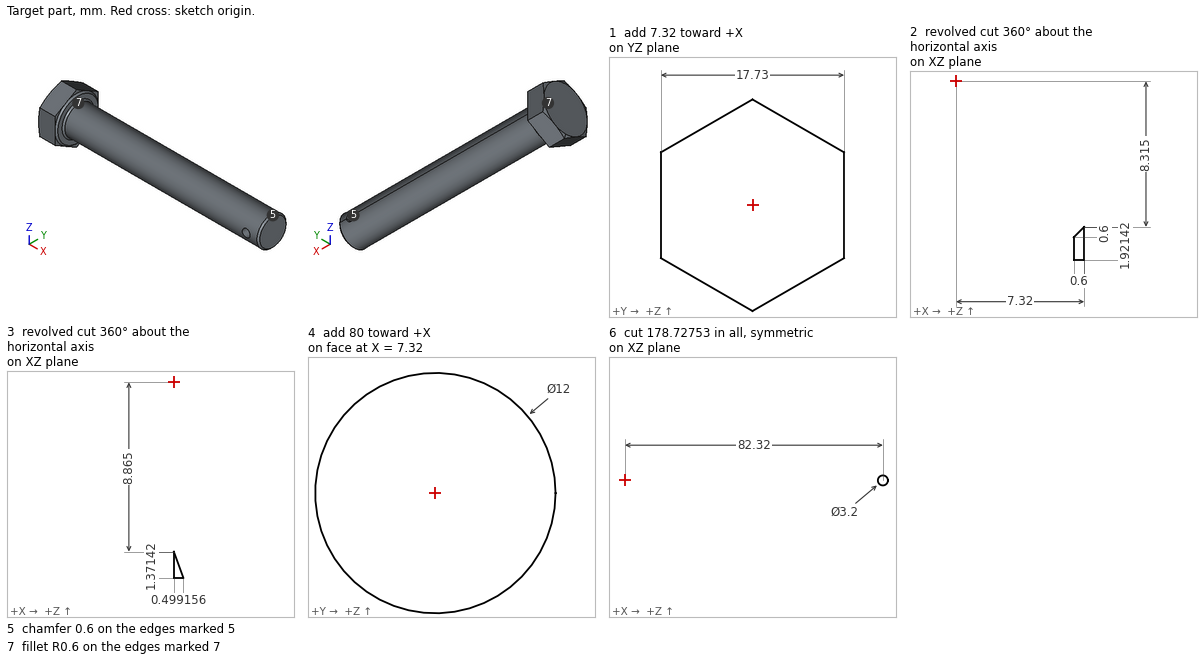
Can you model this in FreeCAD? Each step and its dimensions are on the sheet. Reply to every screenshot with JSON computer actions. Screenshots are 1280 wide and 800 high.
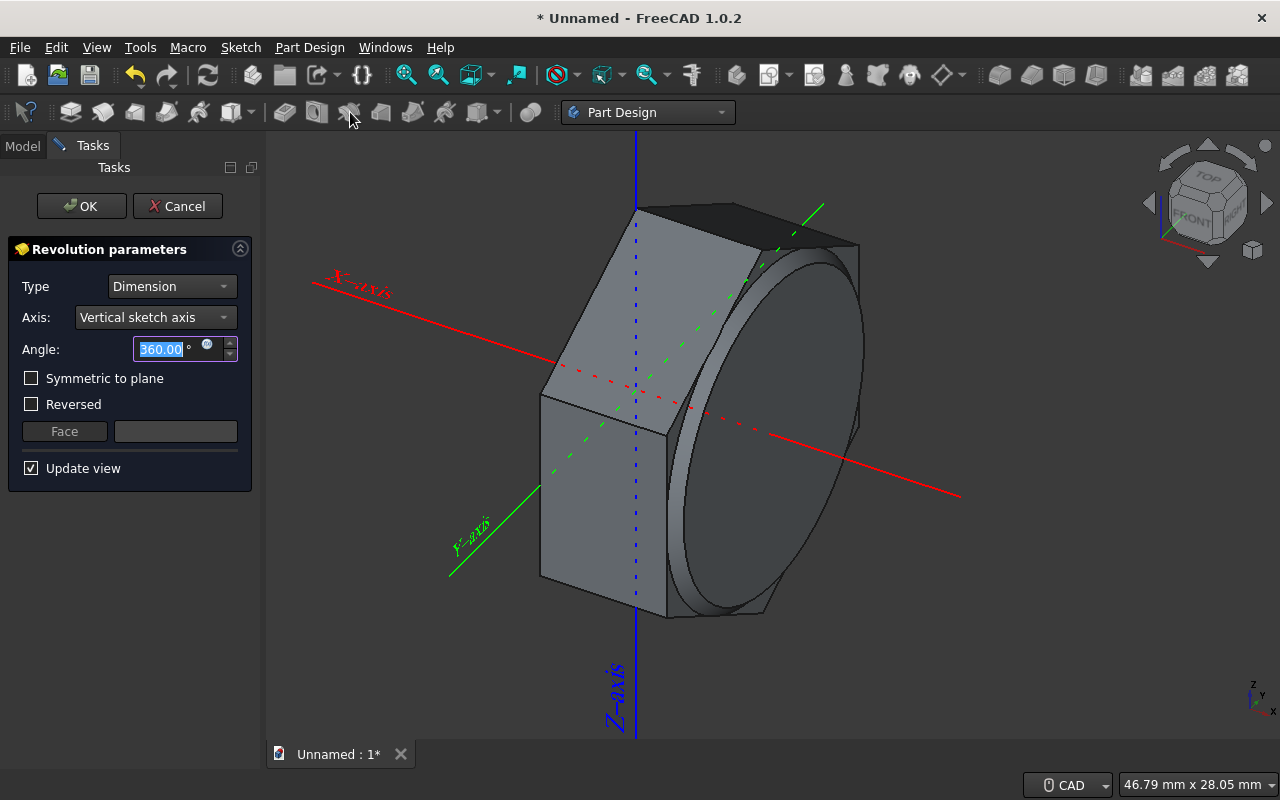
{"action": "left_click", "coordinate": [156, 318]}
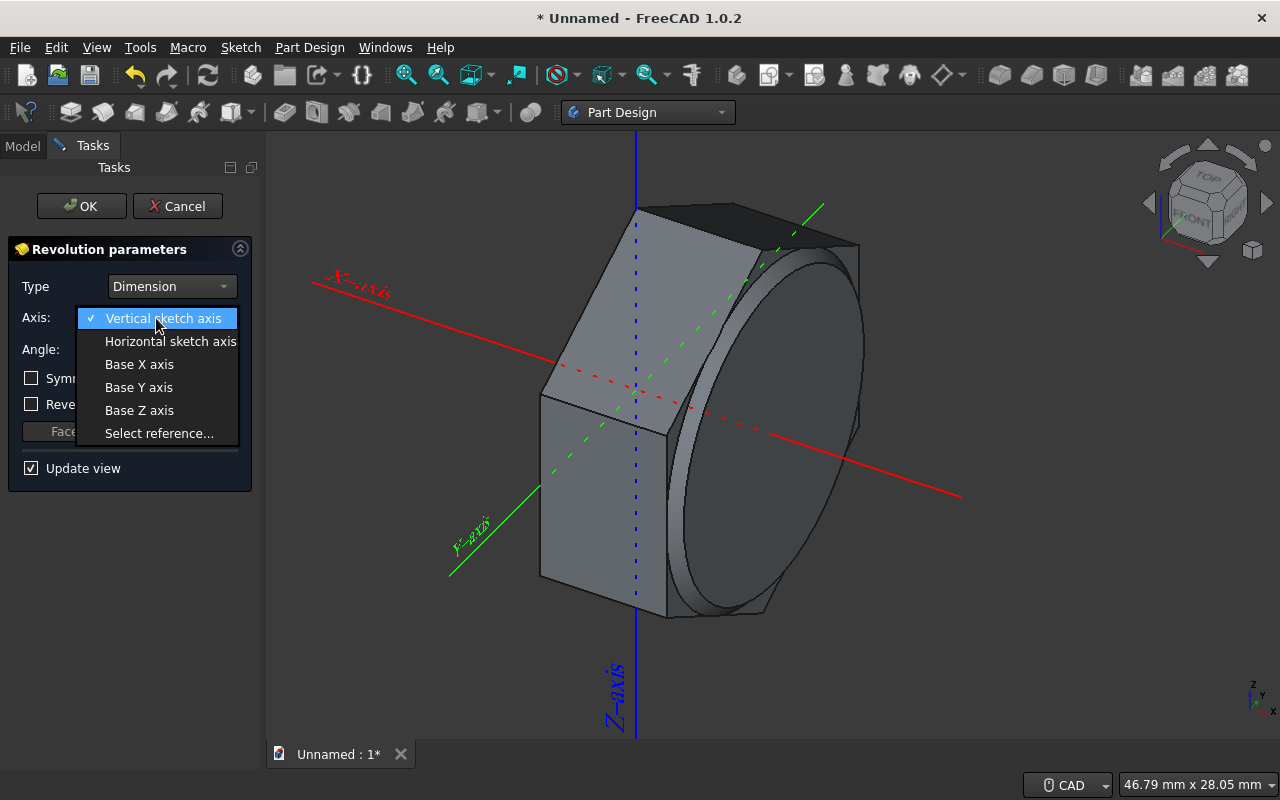
{"action": "left_click", "coordinate": [156, 342]}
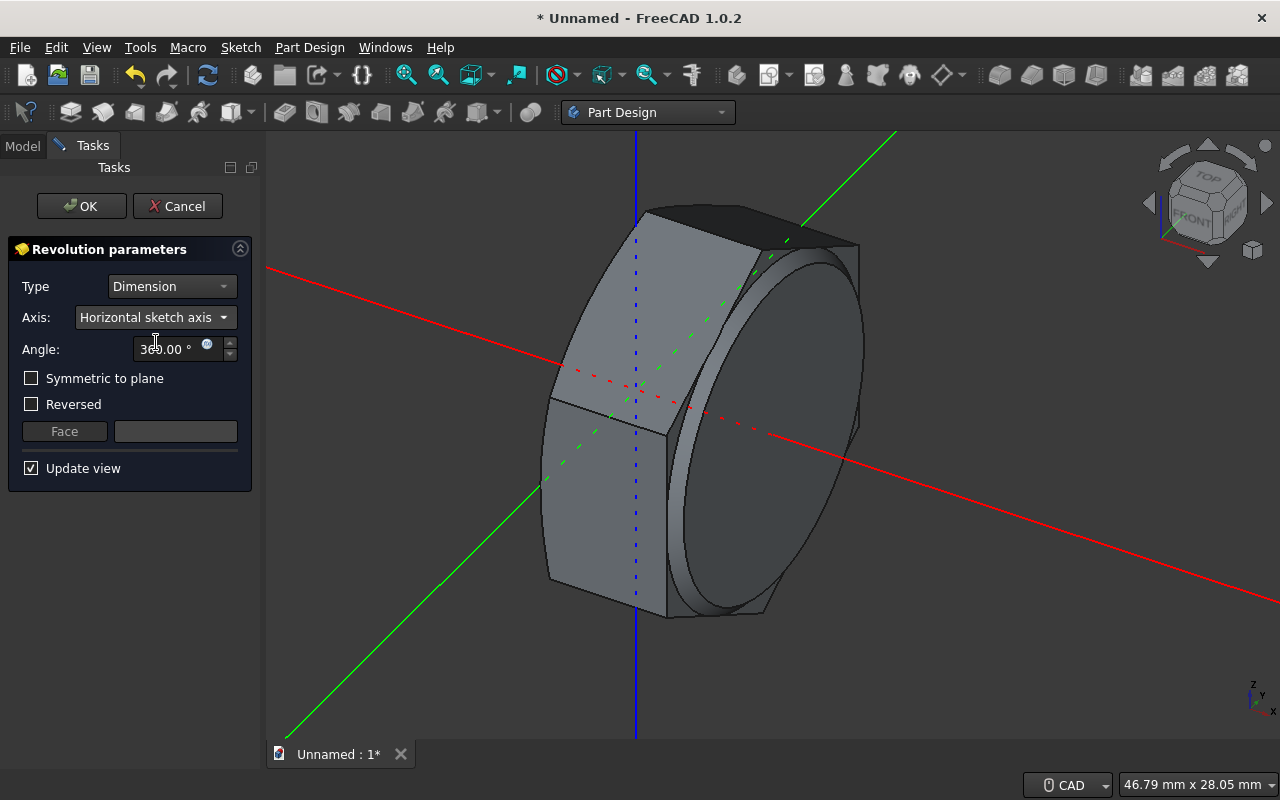
{"action": "left_click", "coordinate": [82, 206]}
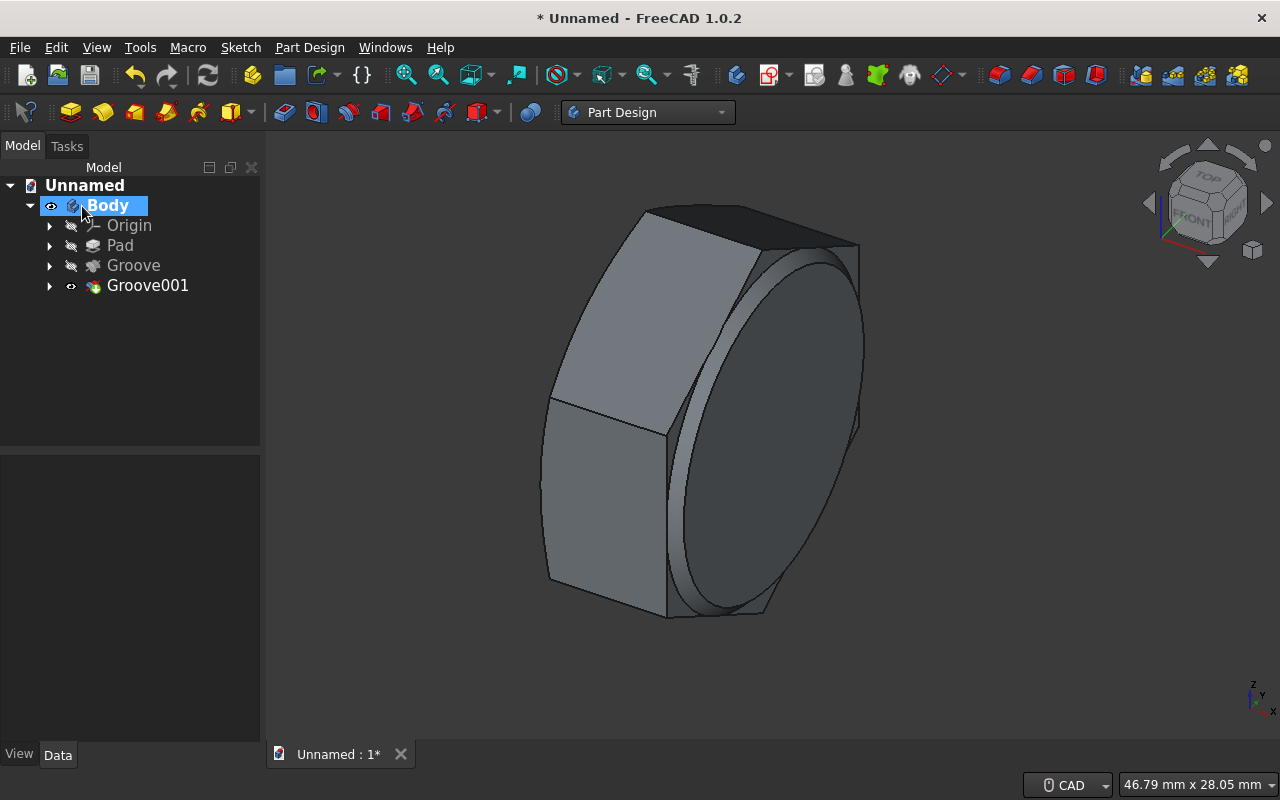
{"action": "left_click", "coordinate": [408, 76]}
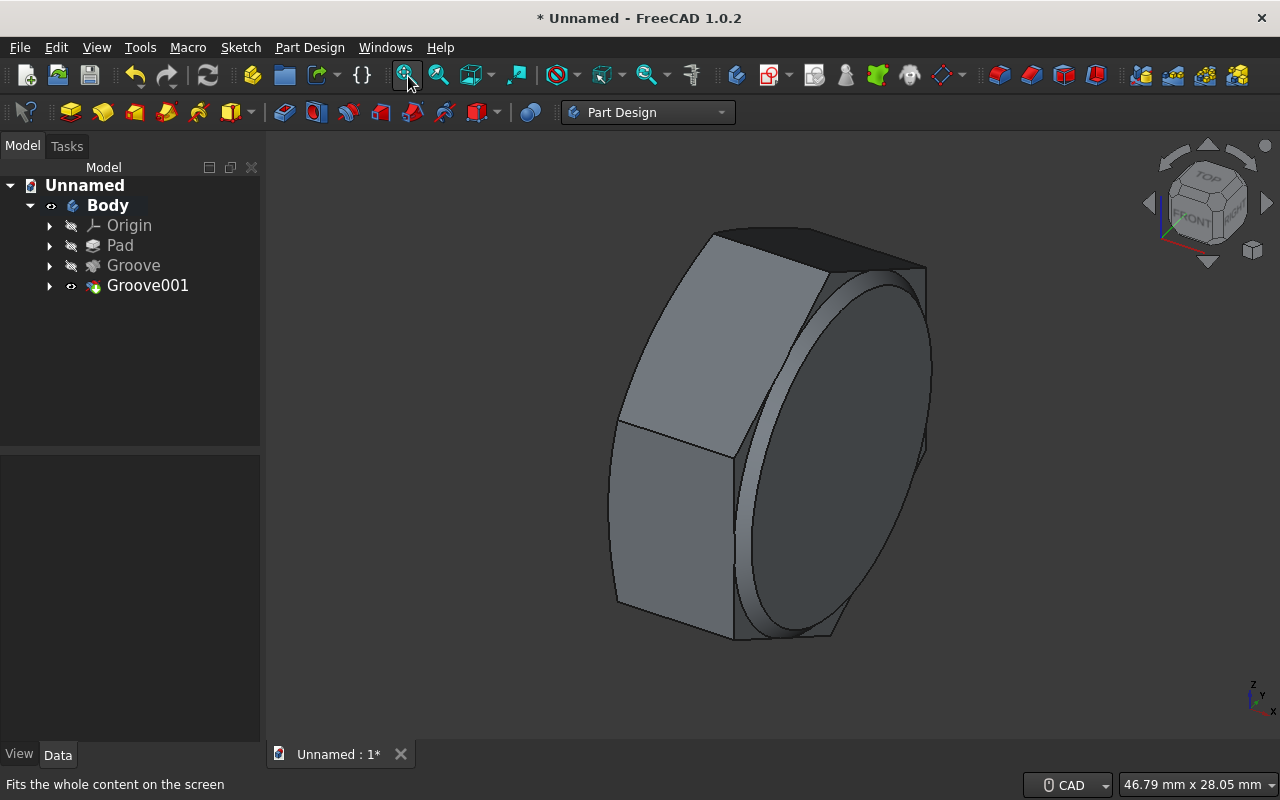
{"action": "left_click", "coordinate": [842, 457]}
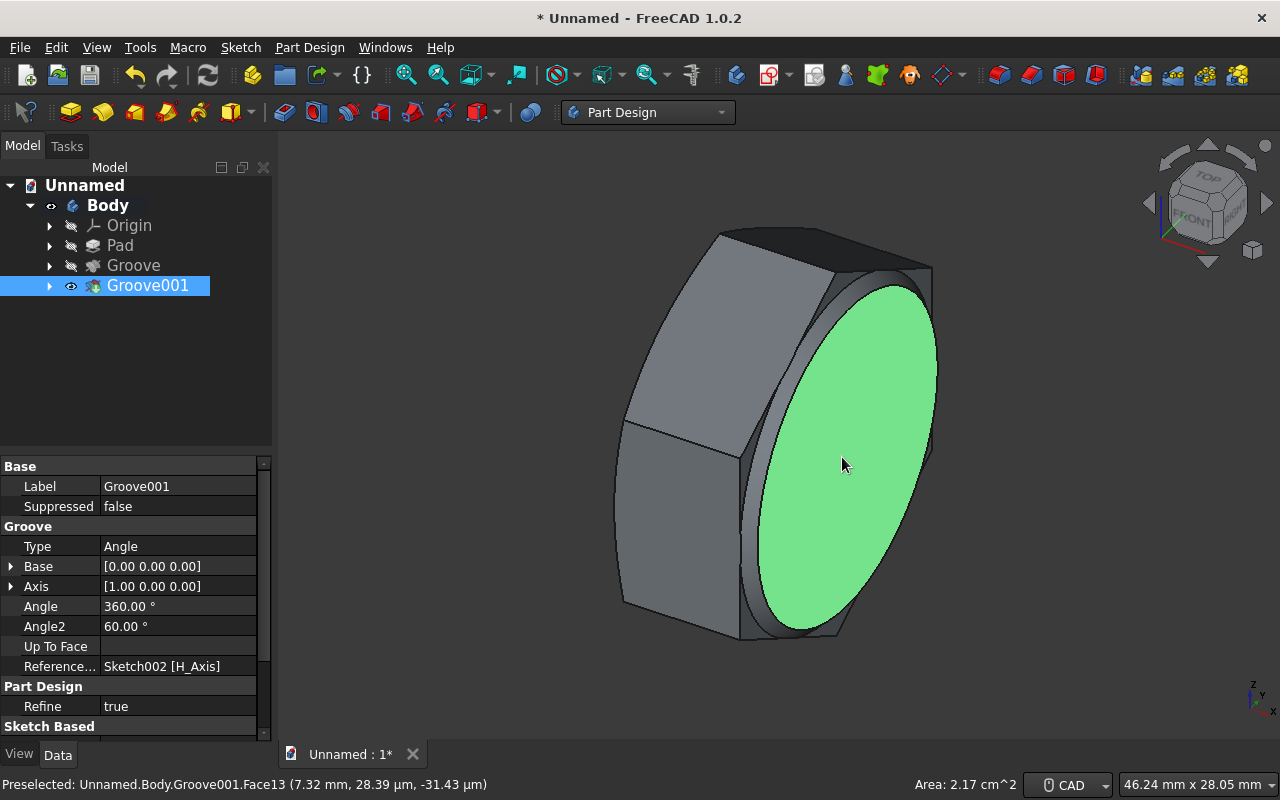
{"action": "left_click", "coordinate": [770, 76]}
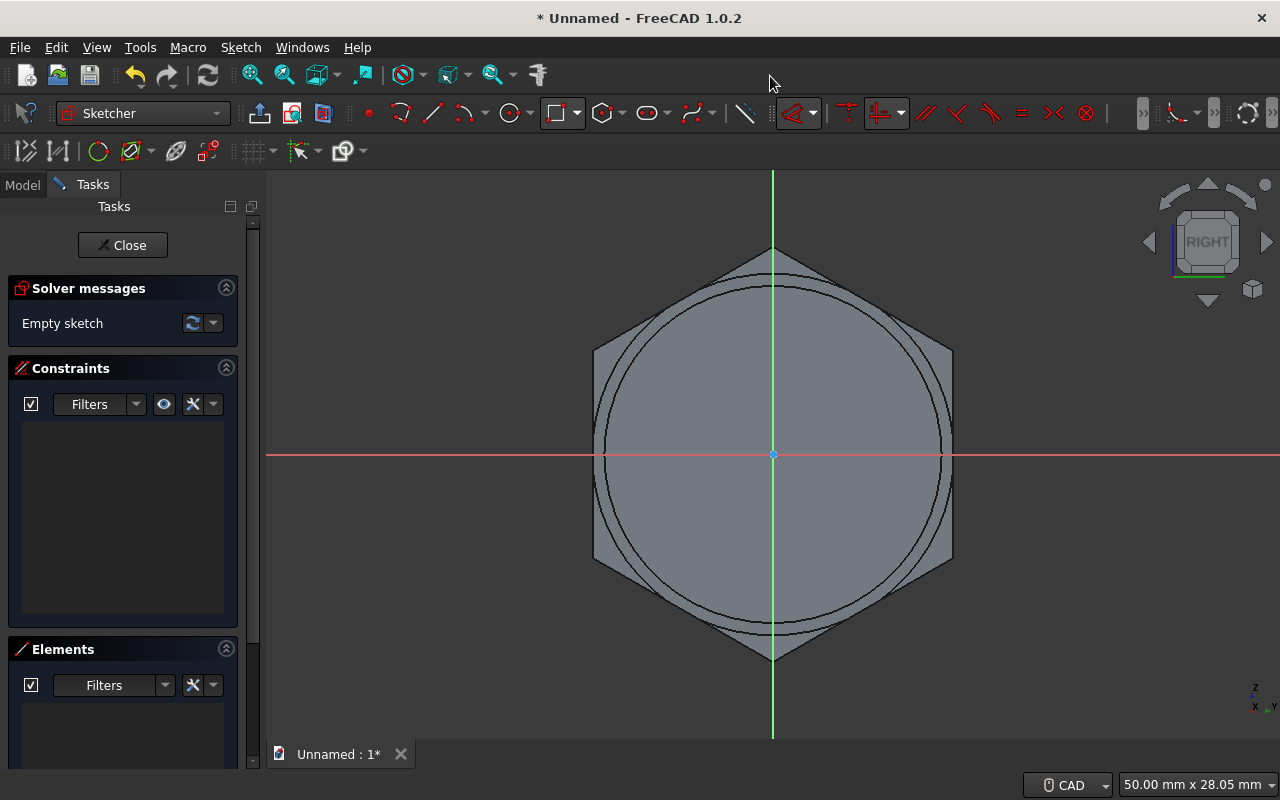
{"action": "scroll", "coordinate": [912, 455], "scroll_direction": "up", "scroll_amount": 2}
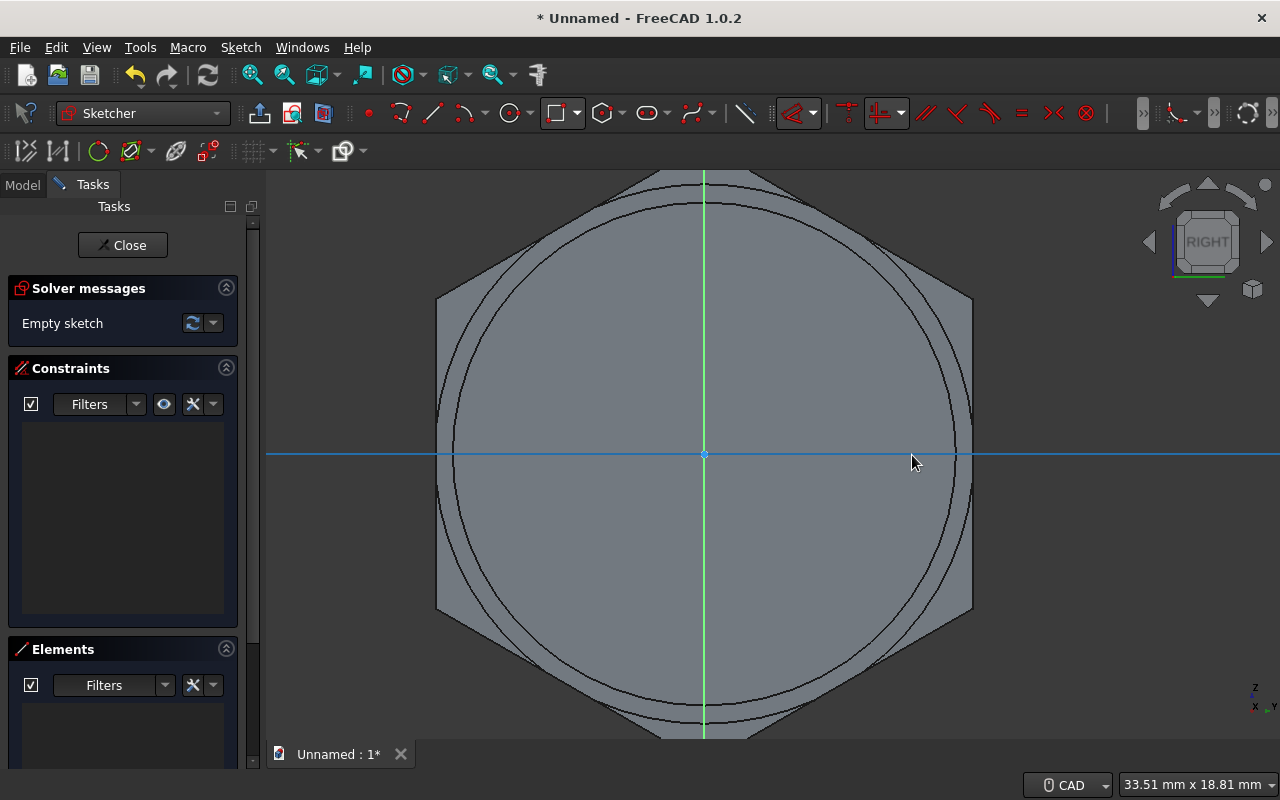
{"action": "left_click", "coordinate": [510, 114]}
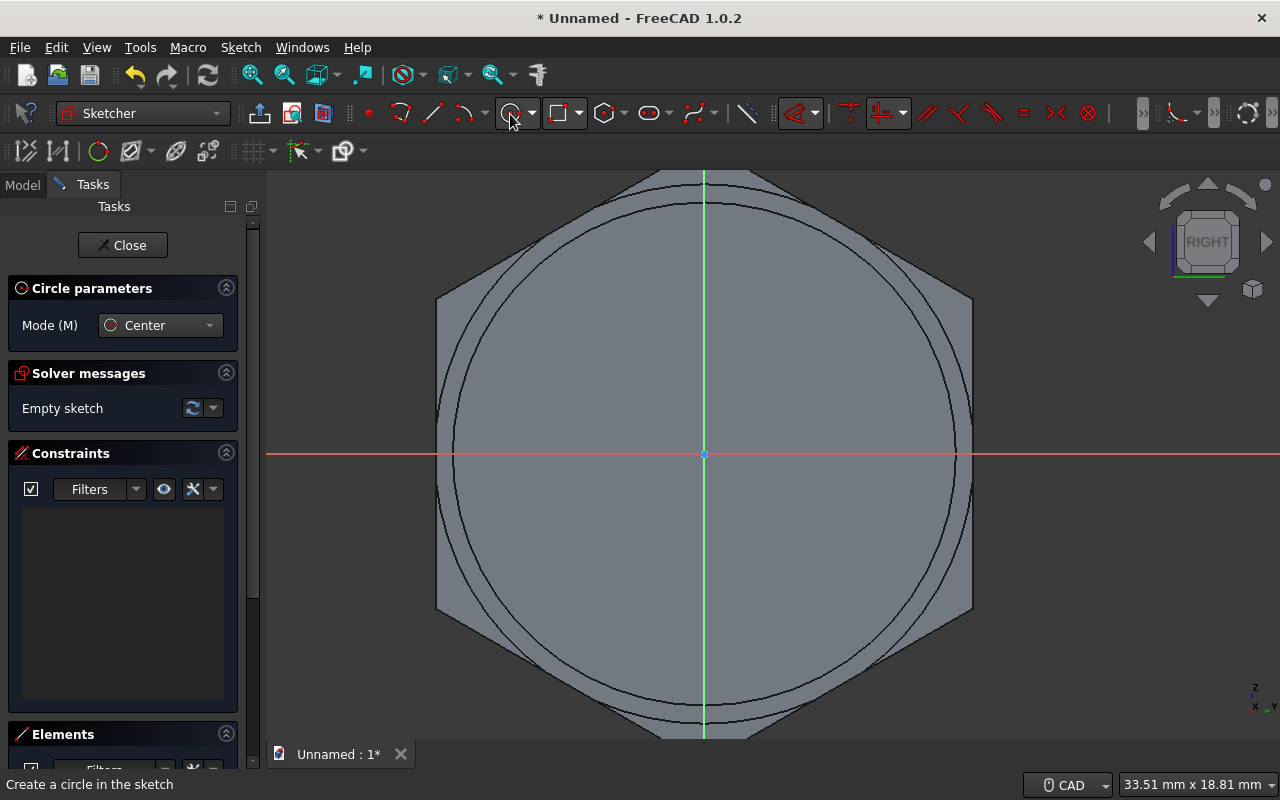
{"action": "left_click", "coordinate": [704, 454]}
{"action": "left_click", "coordinate": [833, 326]}
{"action": "key", "text": "Escape"}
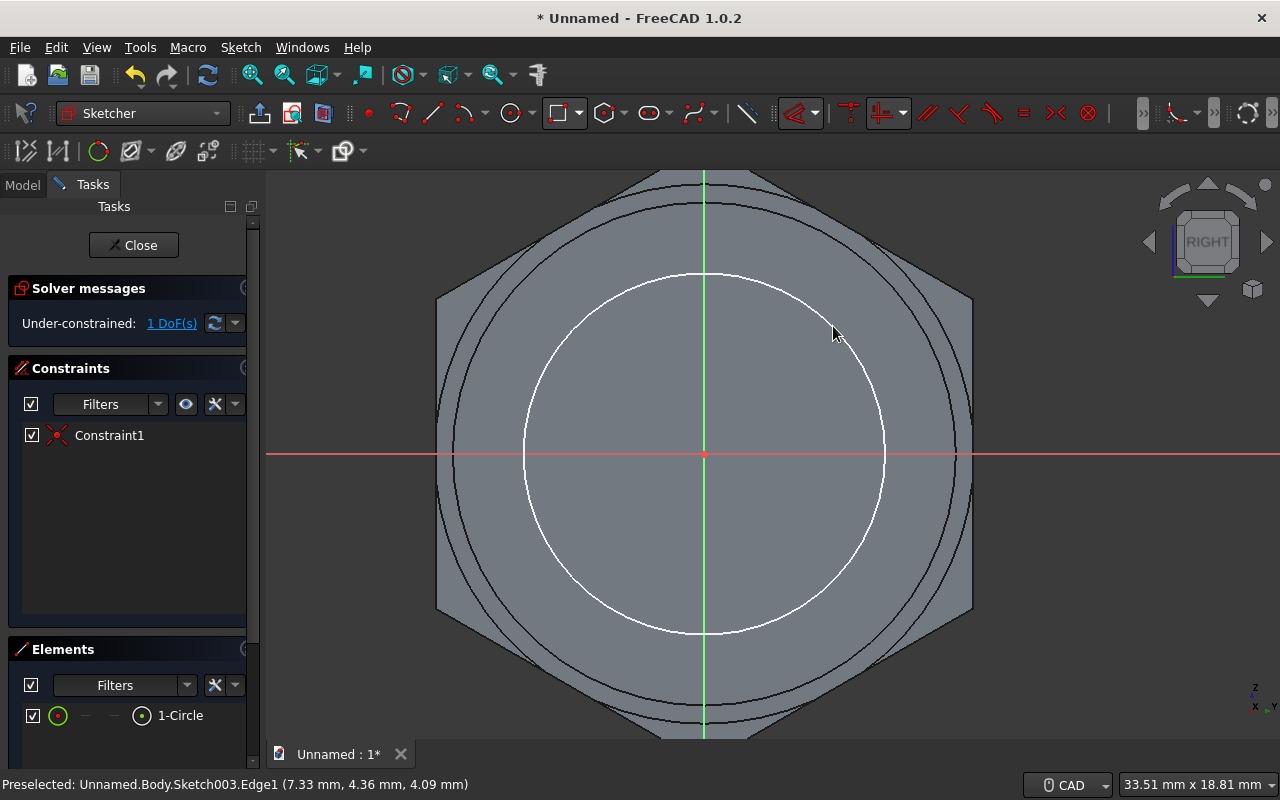
{"action": "left_click", "coordinate": [832, 326]}